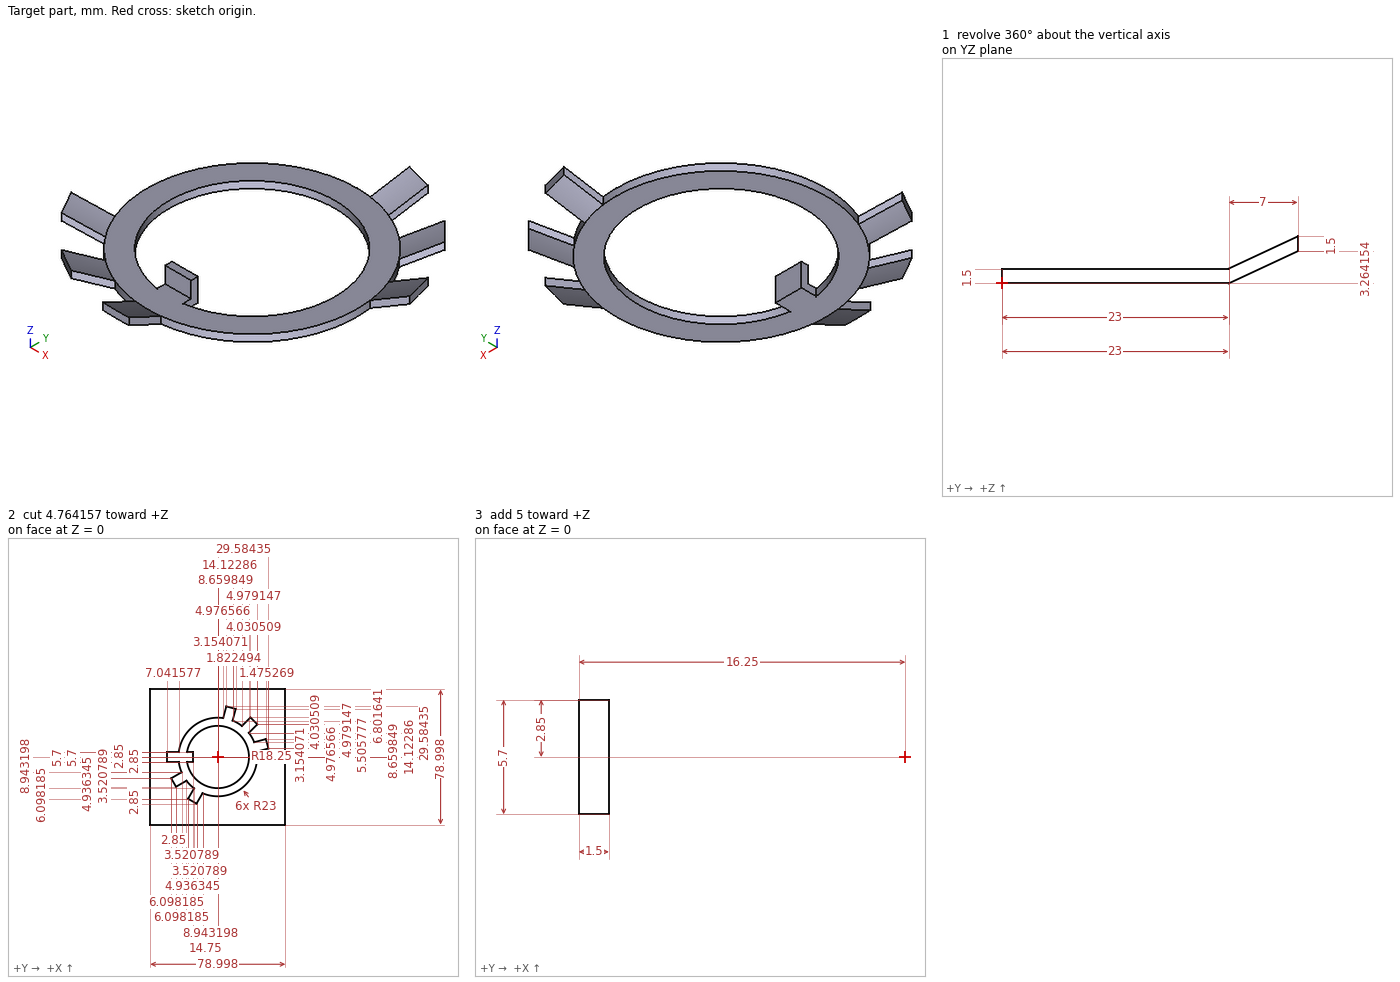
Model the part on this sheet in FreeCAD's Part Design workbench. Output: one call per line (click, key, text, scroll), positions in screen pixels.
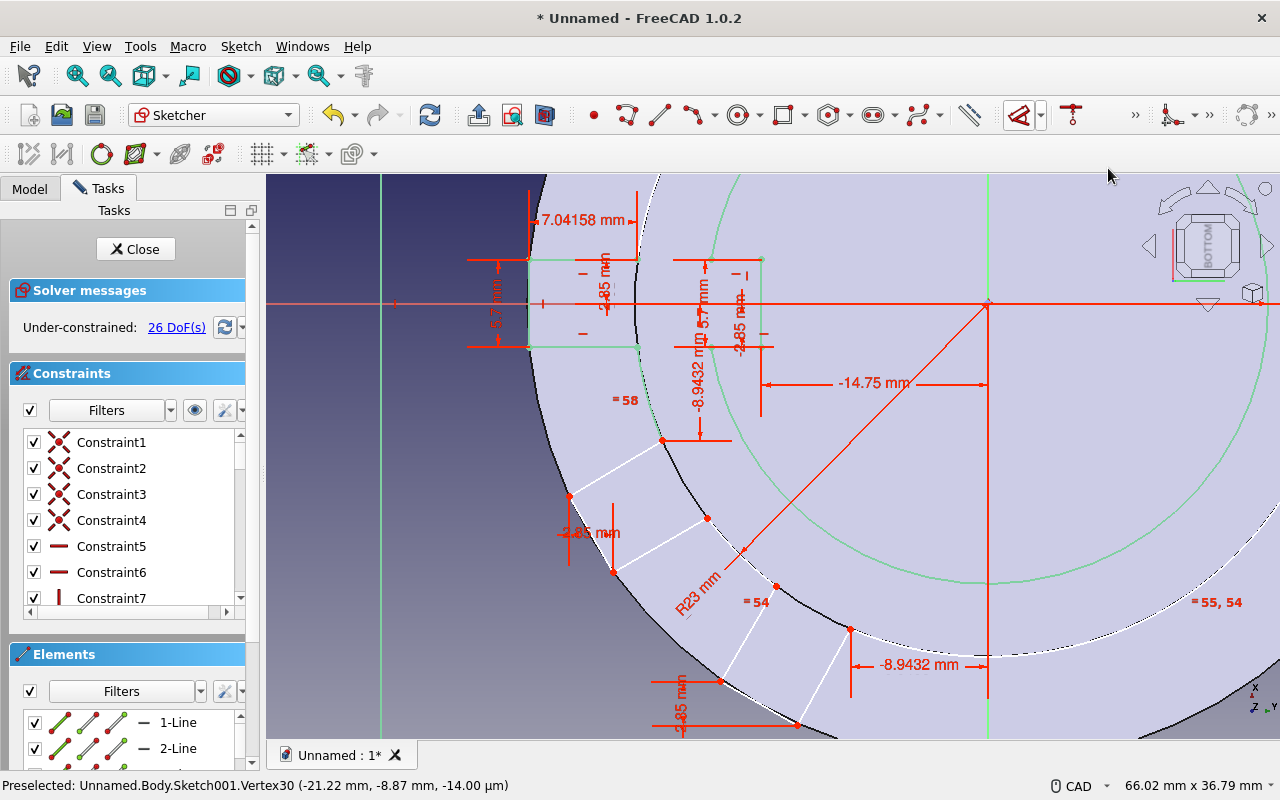
scroll(582, 522, down, 6)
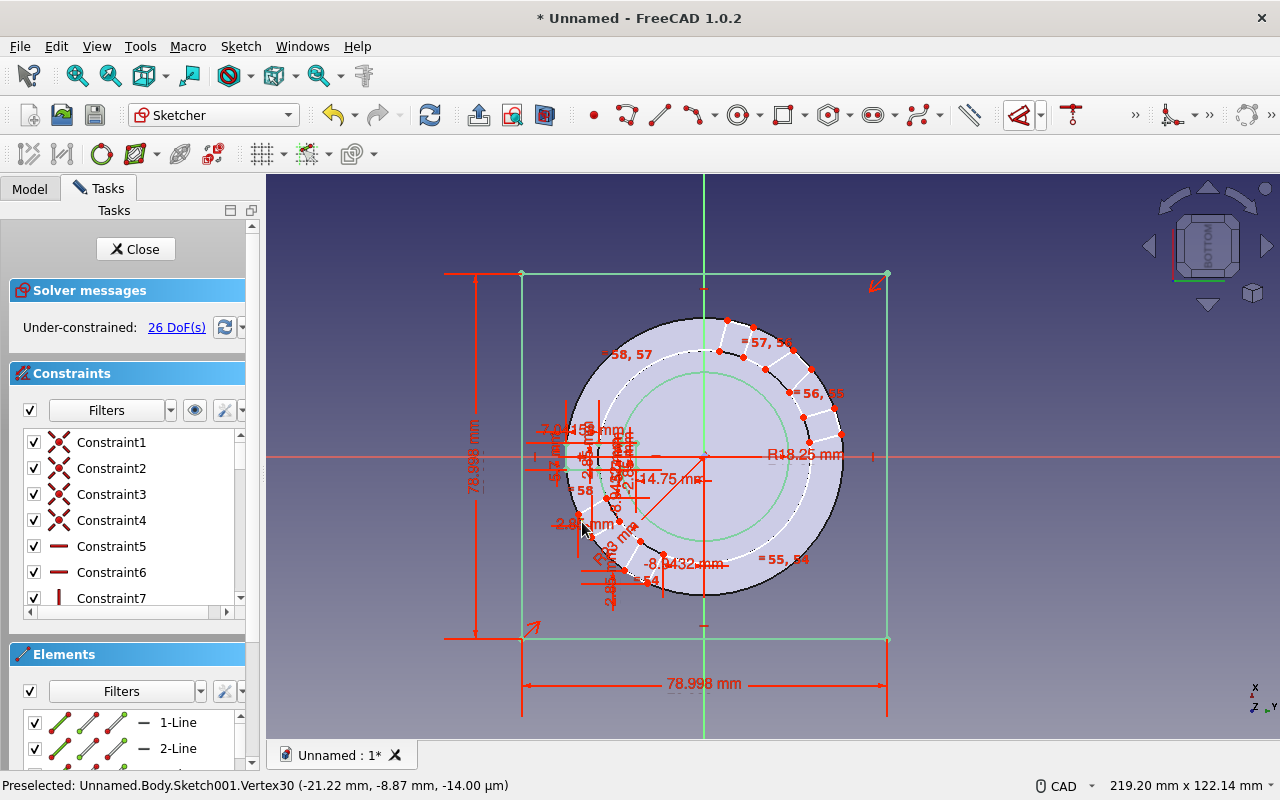
scroll(810, 443, up, 6)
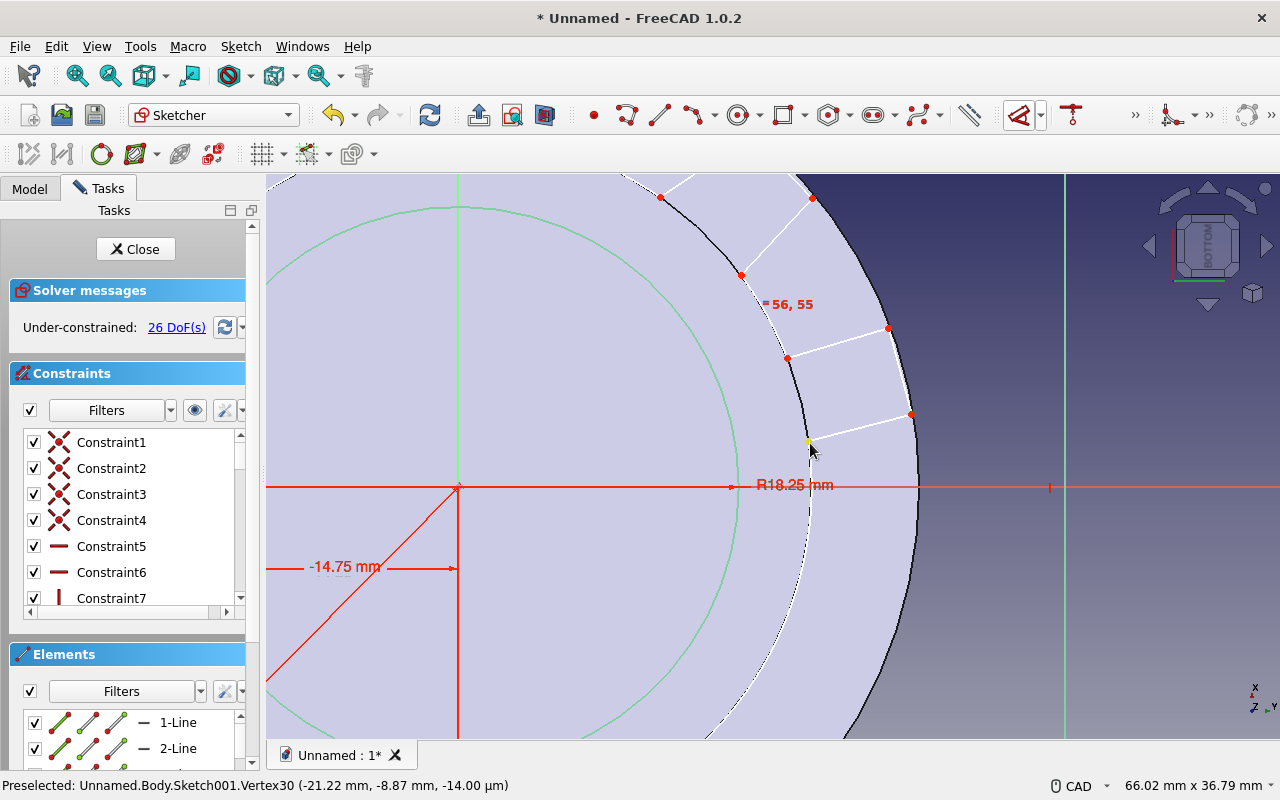
click(809, 441)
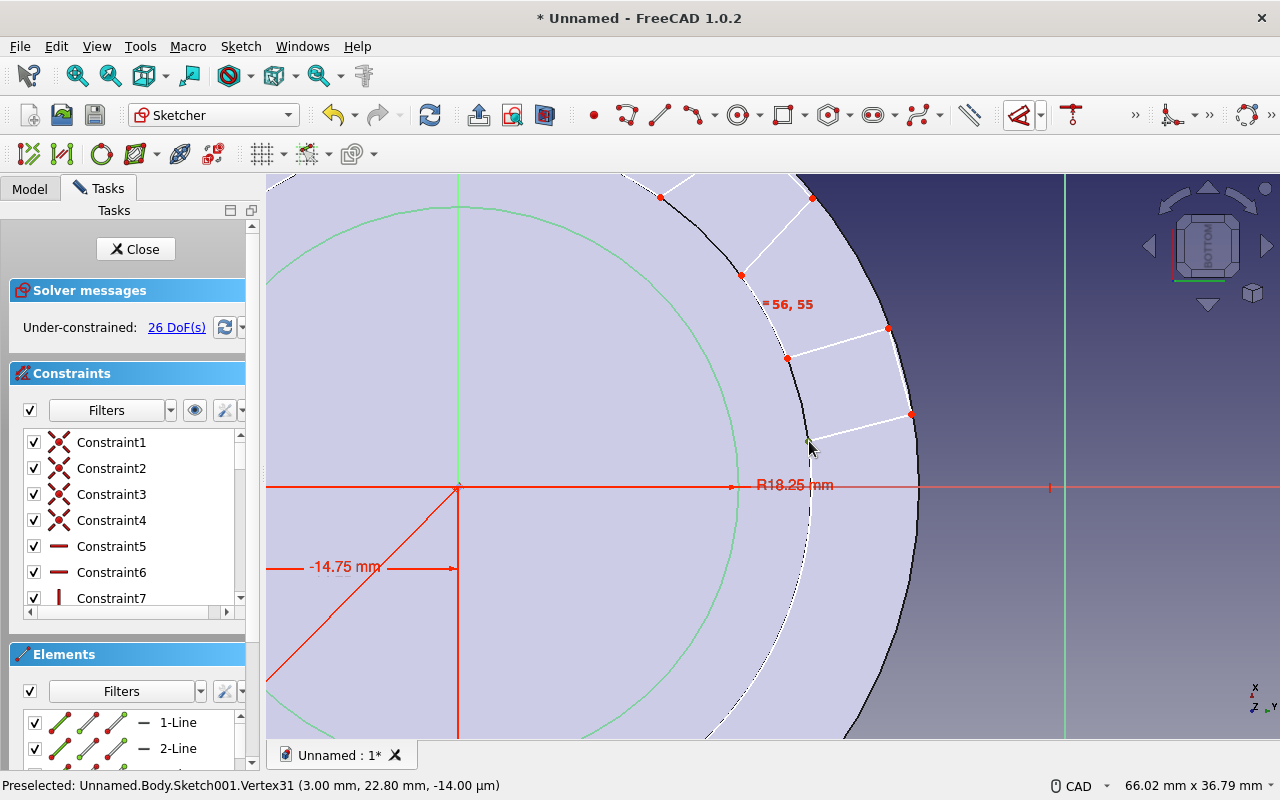
click(1040, 116)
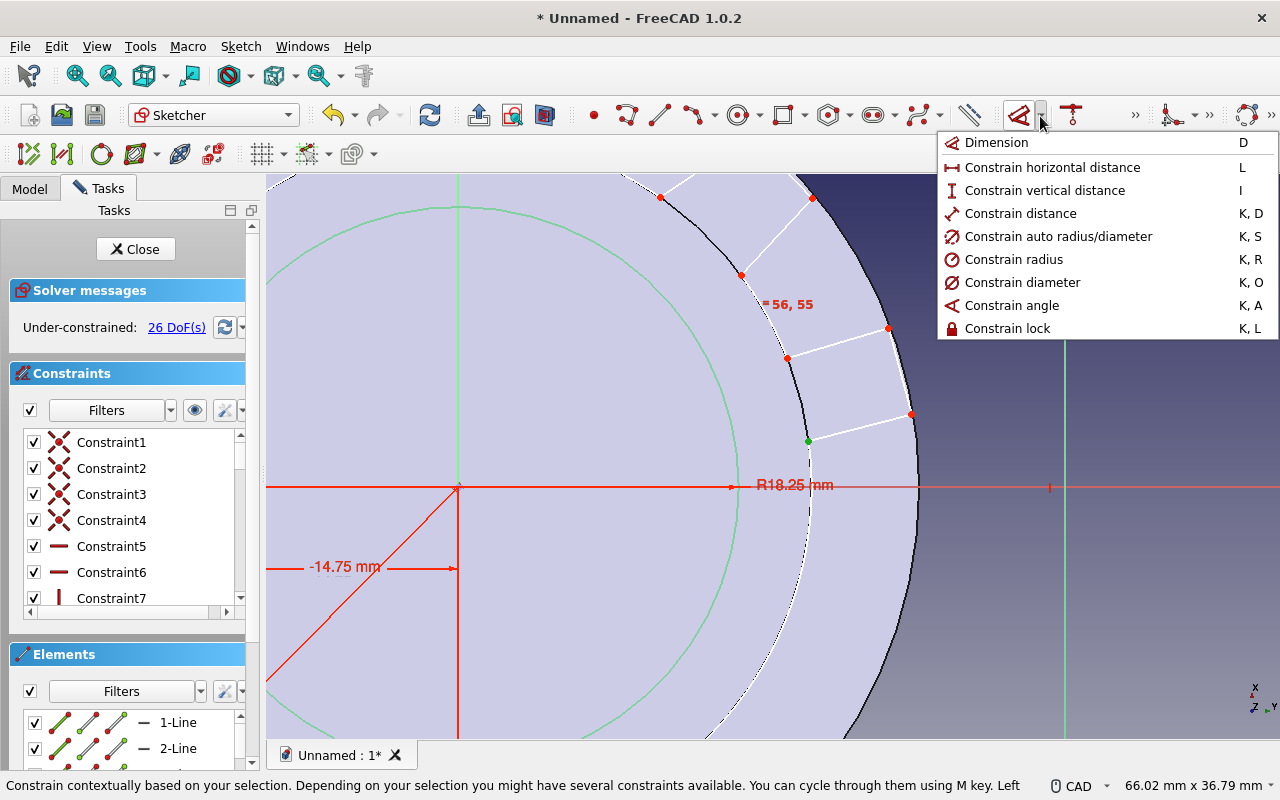
click(1108, 190)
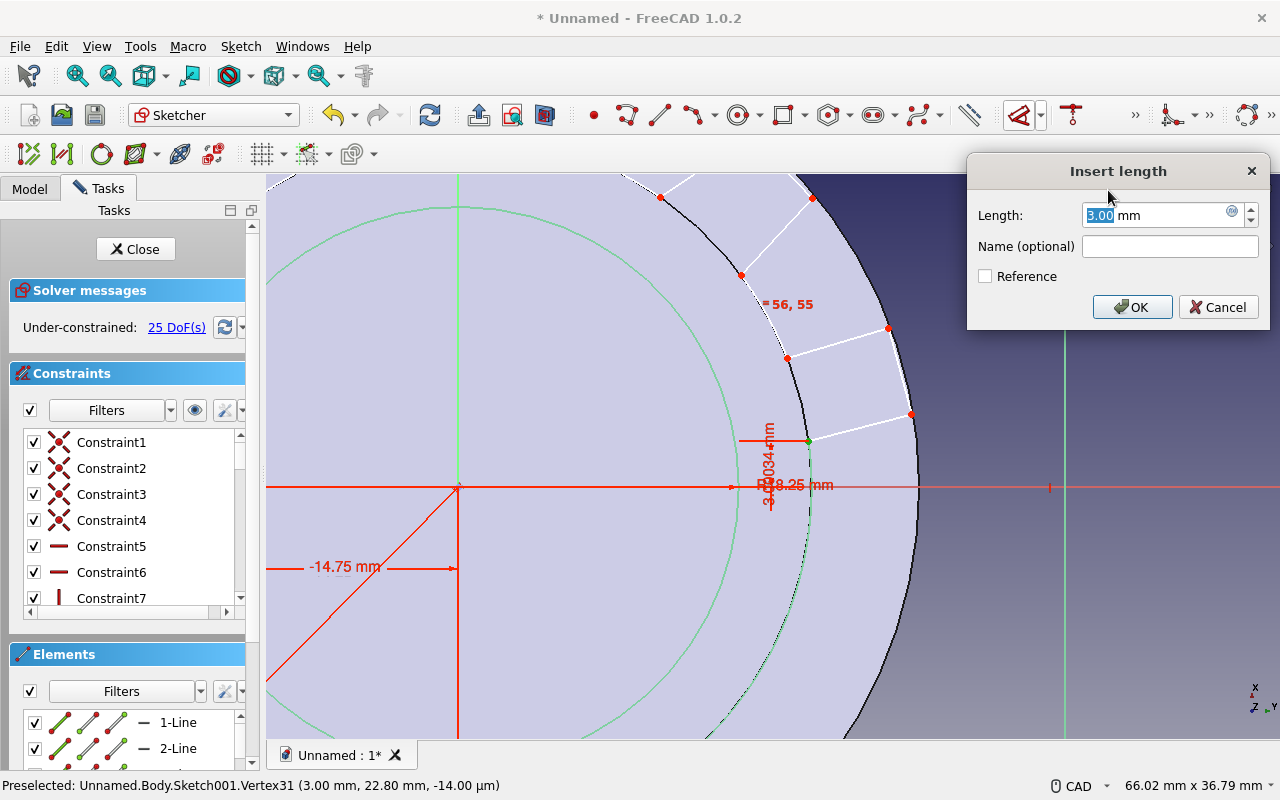
text(3.154071)
key(Return)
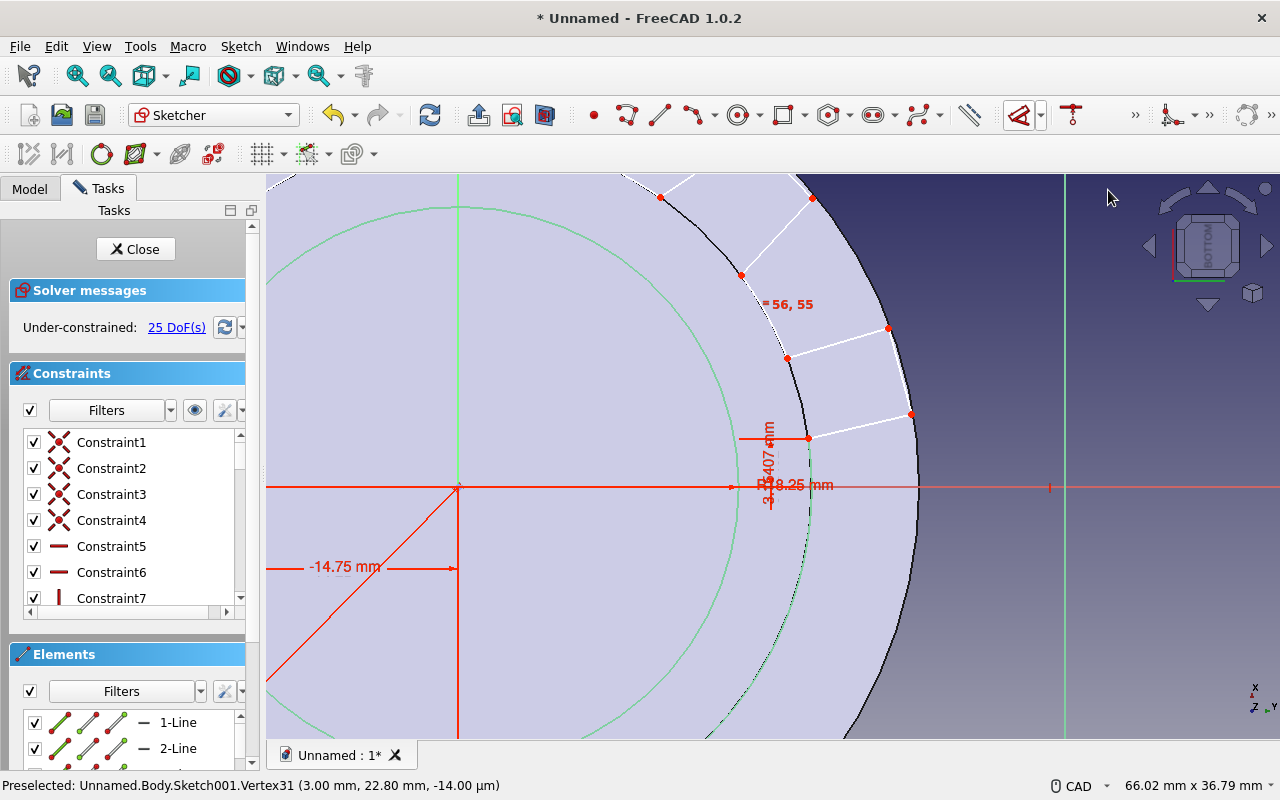
click(912, 414)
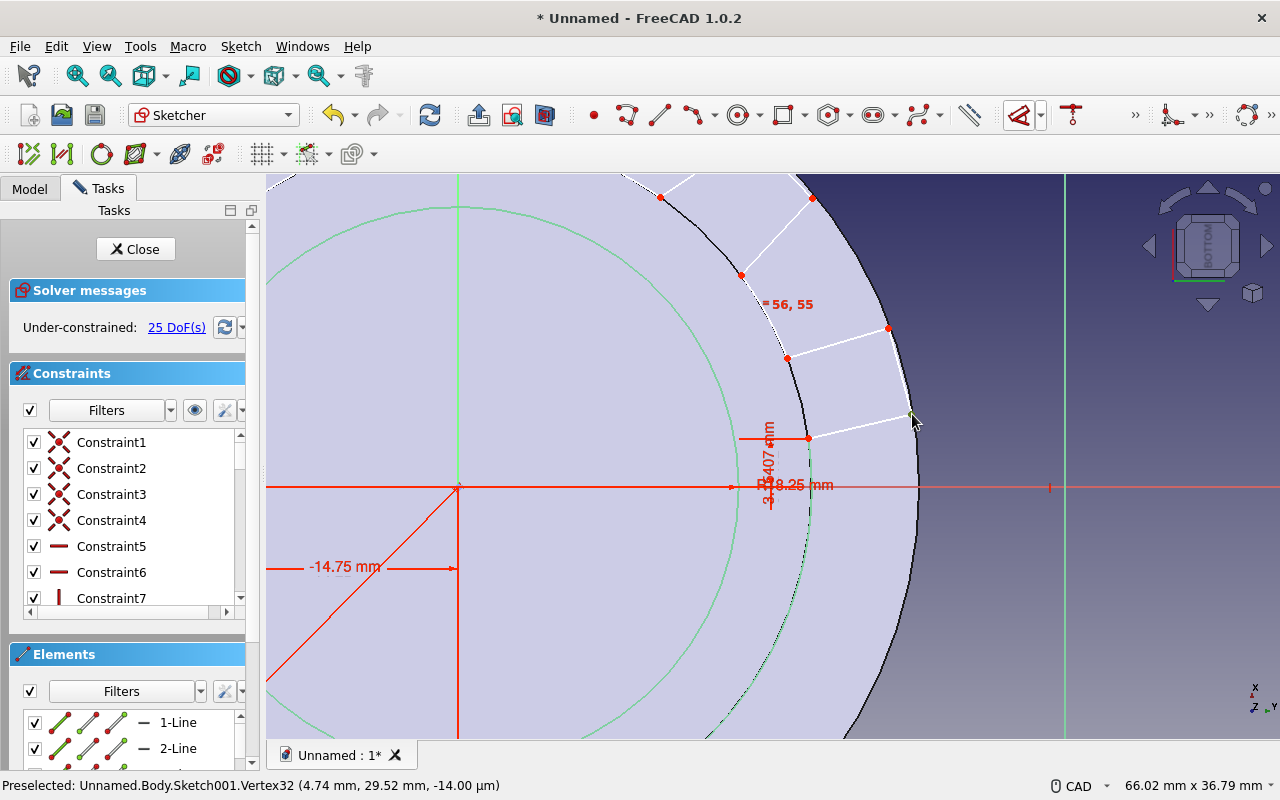
key(l)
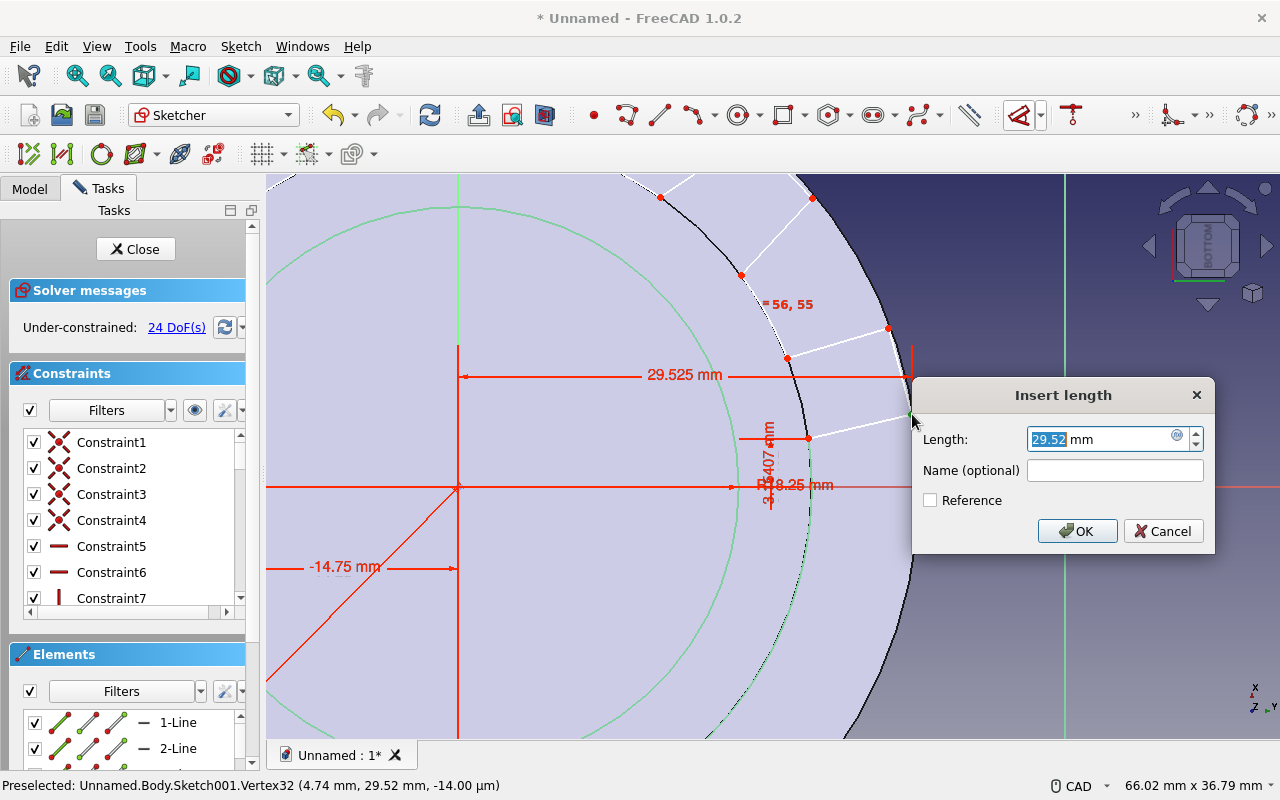
text(29.58435)
key(Return)